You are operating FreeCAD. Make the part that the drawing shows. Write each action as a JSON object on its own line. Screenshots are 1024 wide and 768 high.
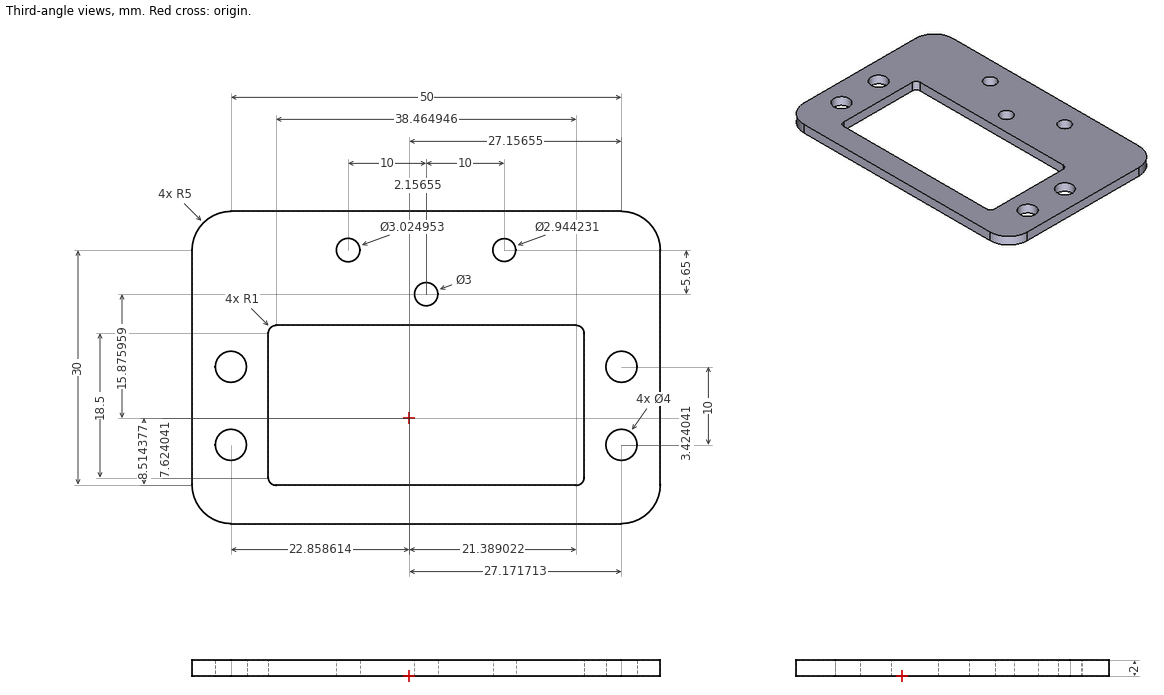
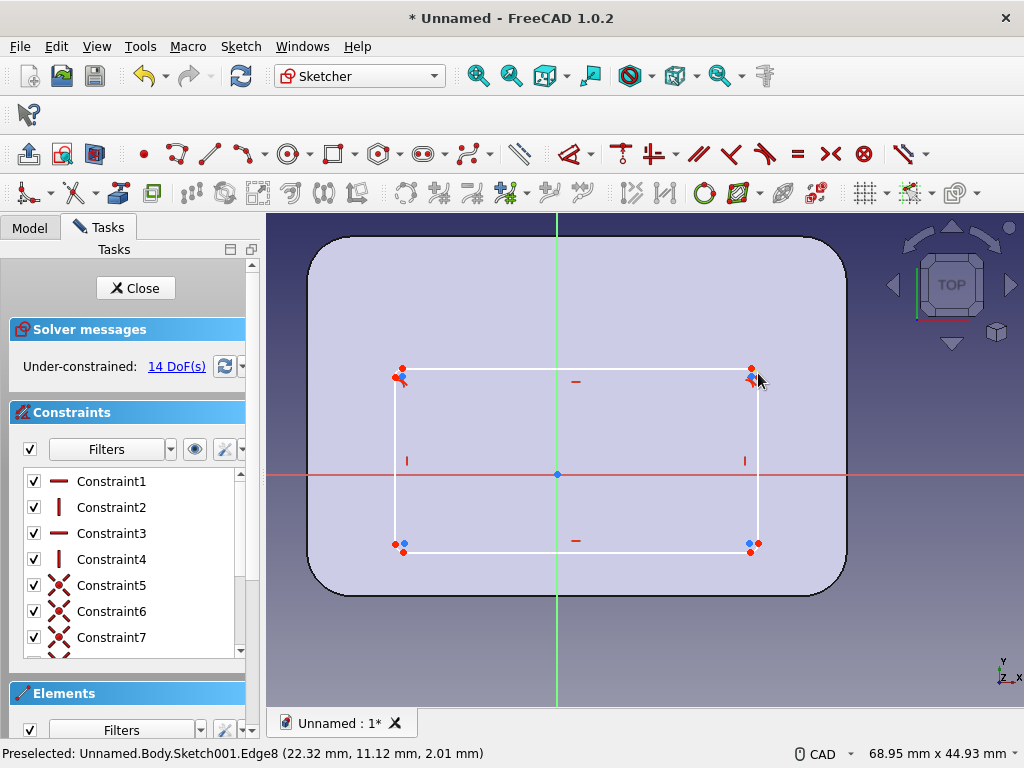
{"action": "left_click", "coordinate": [395, 428]}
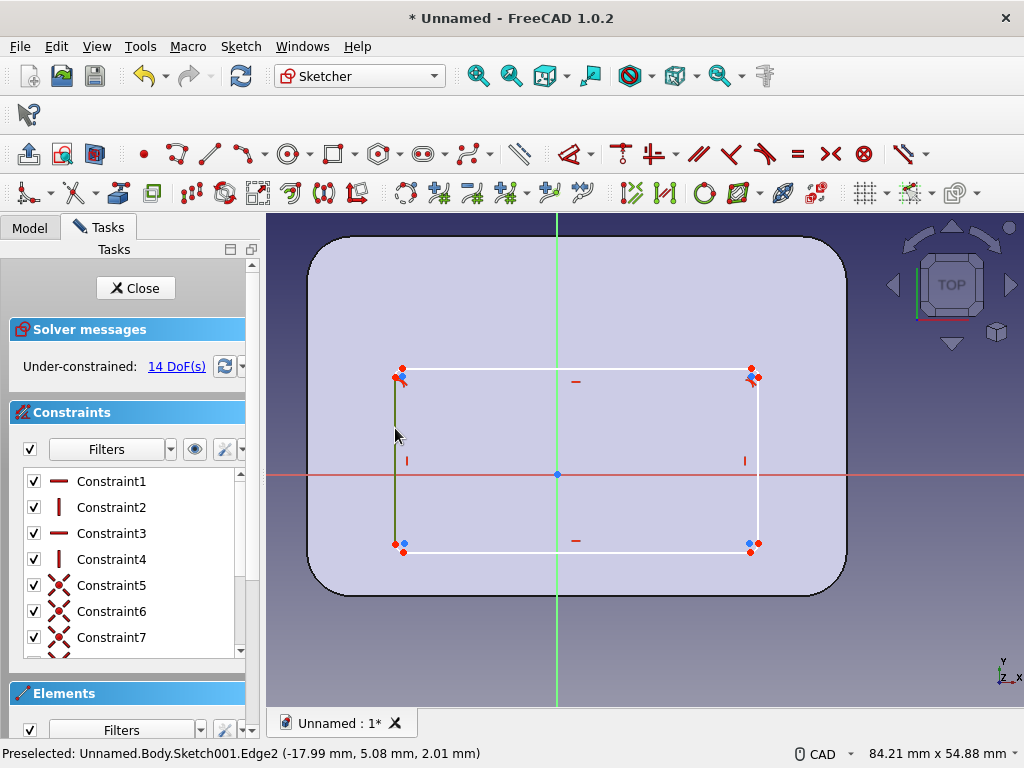
{"action": "scroll", "coordinate": [397, 372], "scroll_direction": "up", "scroll_amount": 4}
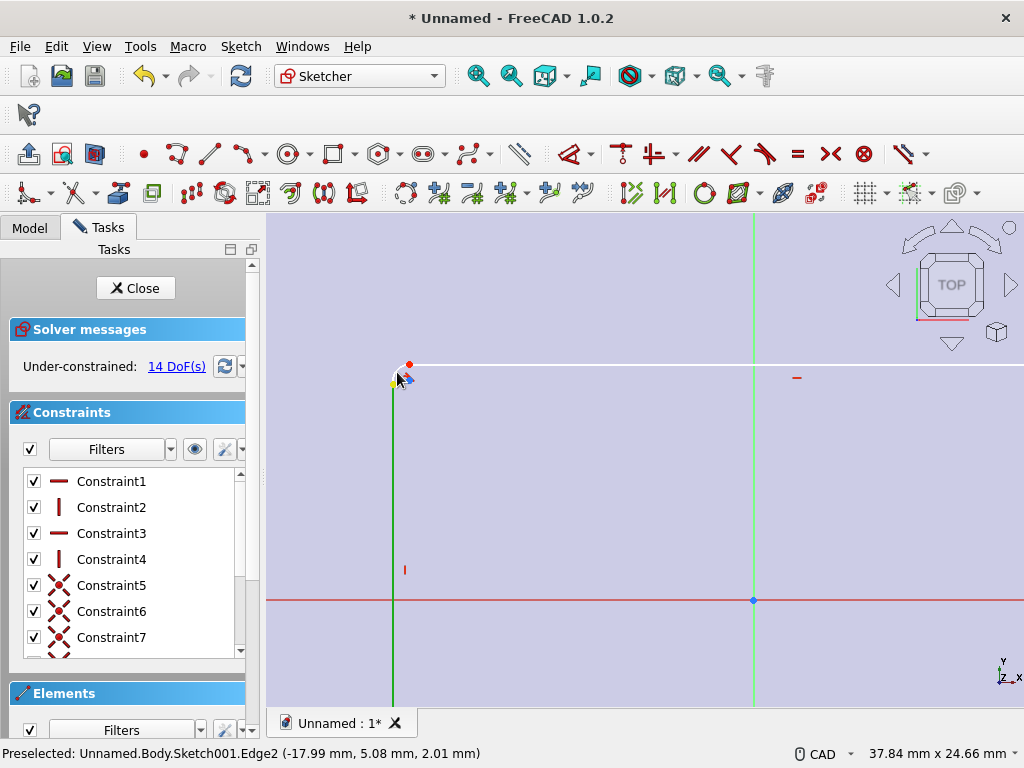
{"action": "left_click", "coordinate": [397, 371]}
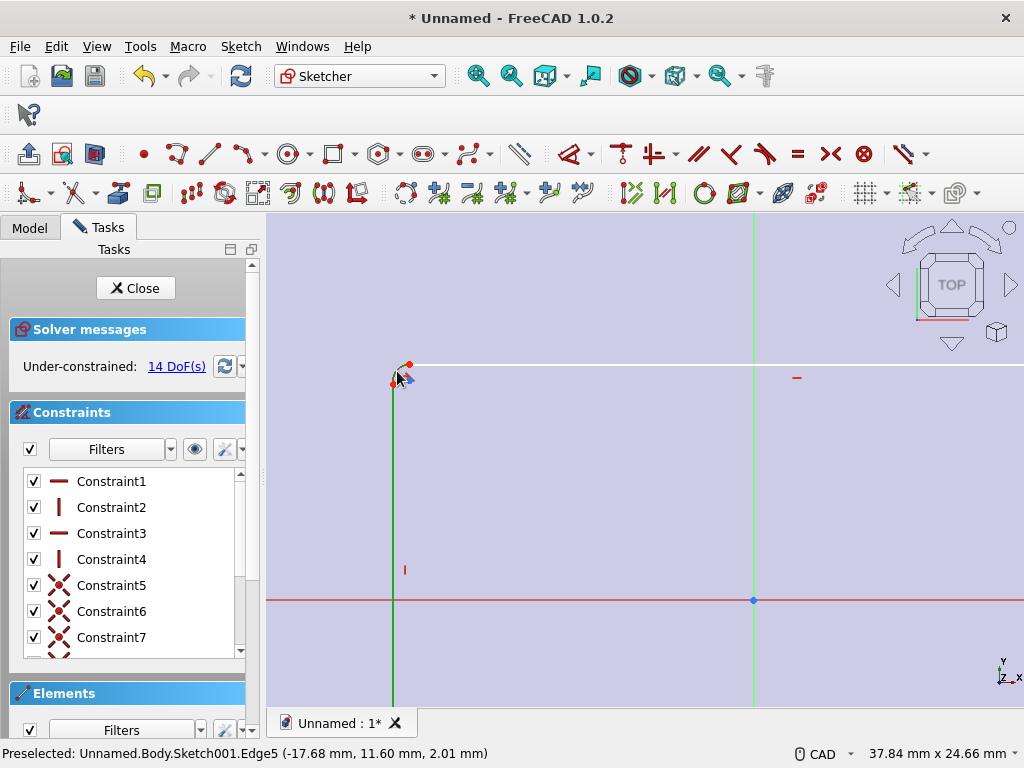
{"action": "left_click", "coordinate": [765, 154]}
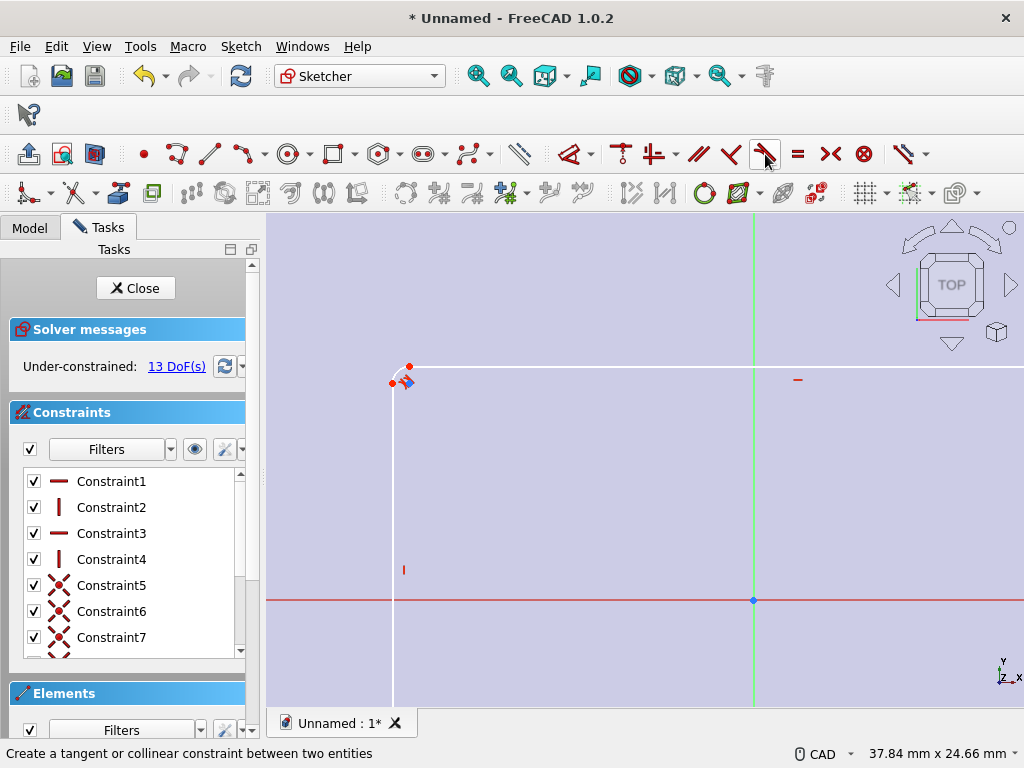
{"action": "left_click", "coordinate": [393, 495]}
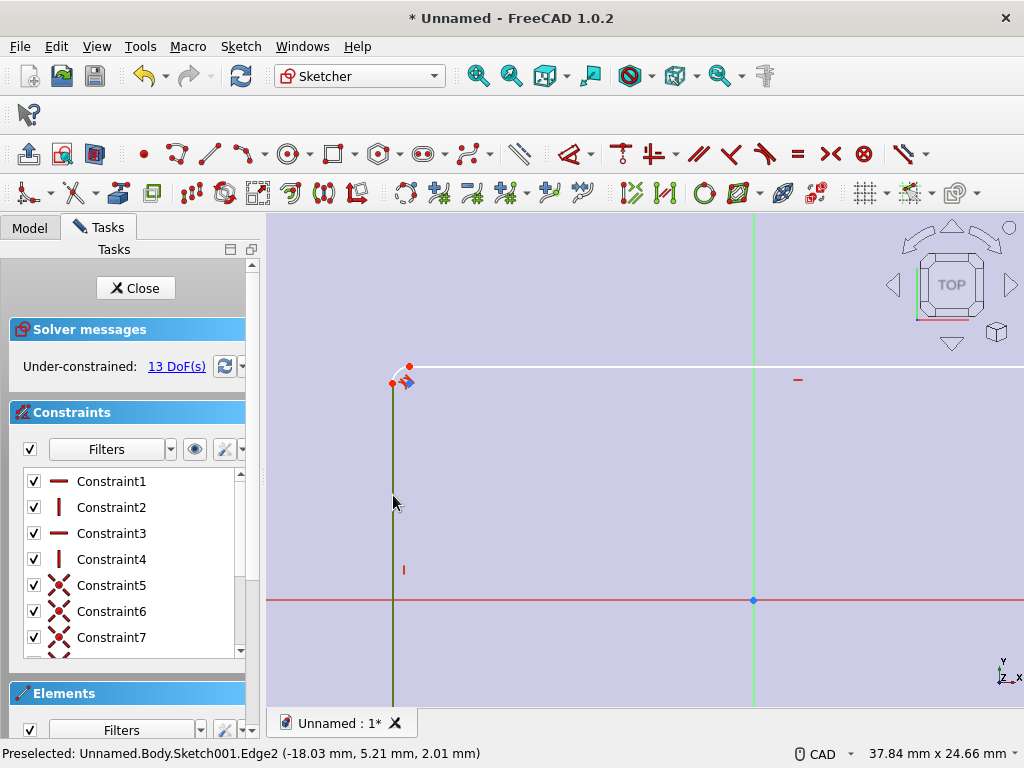
{"action": "scroll", "coordinate": [397, 372], "scroll_direction": "down", "scroll_amount": 4}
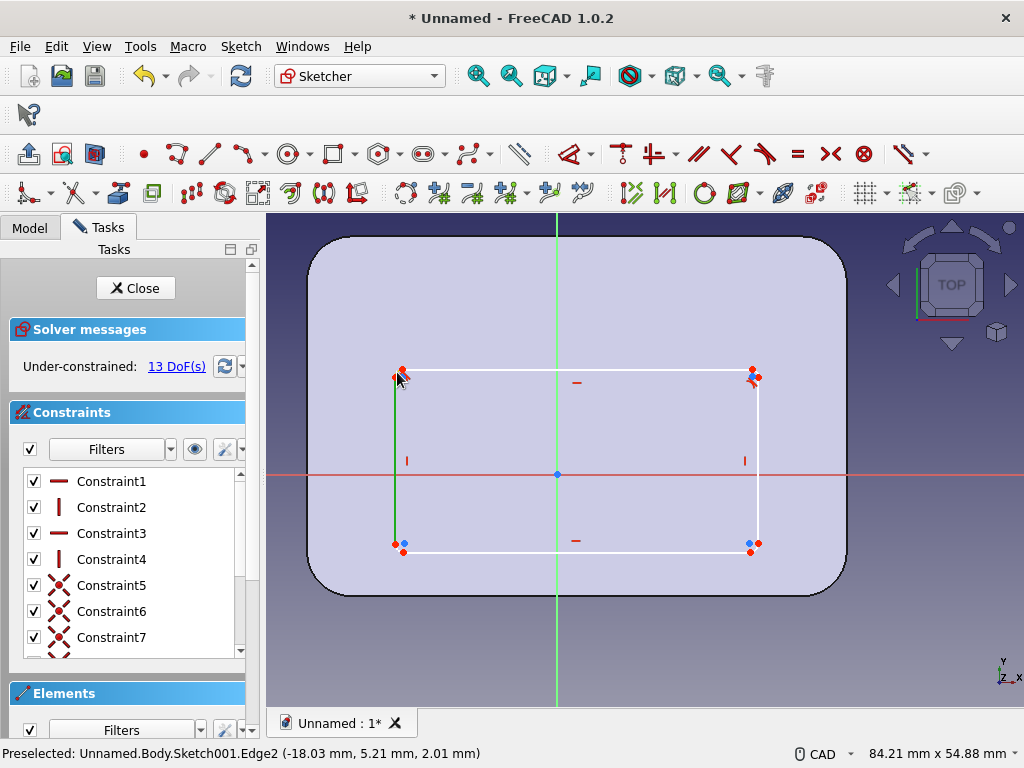
{"action": "scroll", "coordinate": [398, 550], "scroll_direction": "up", "scroll_amount": 5}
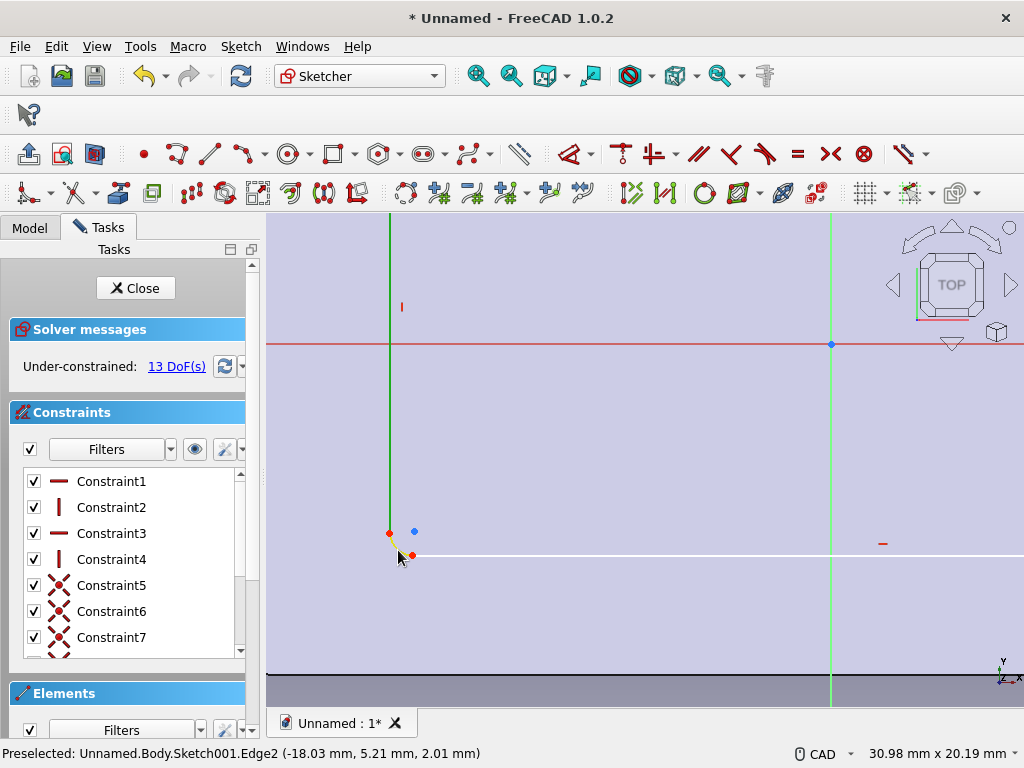
{"action": "left_click", "coordinate": [397, 549]}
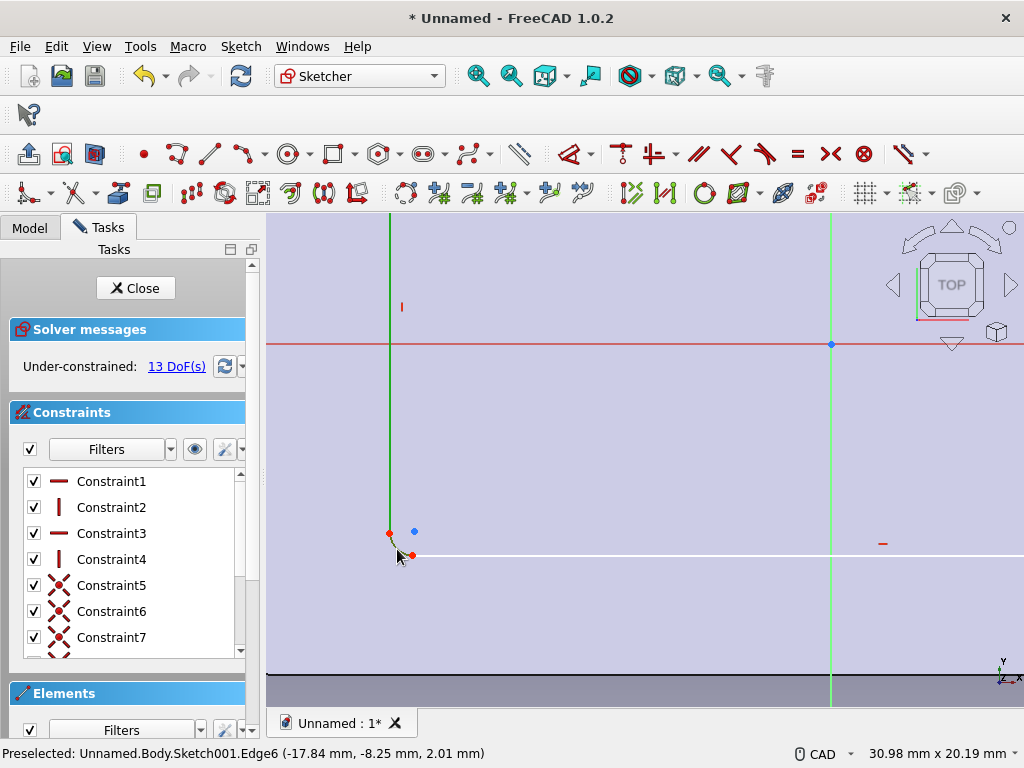
{"action": "left_click", "coordinate": [765, 154]}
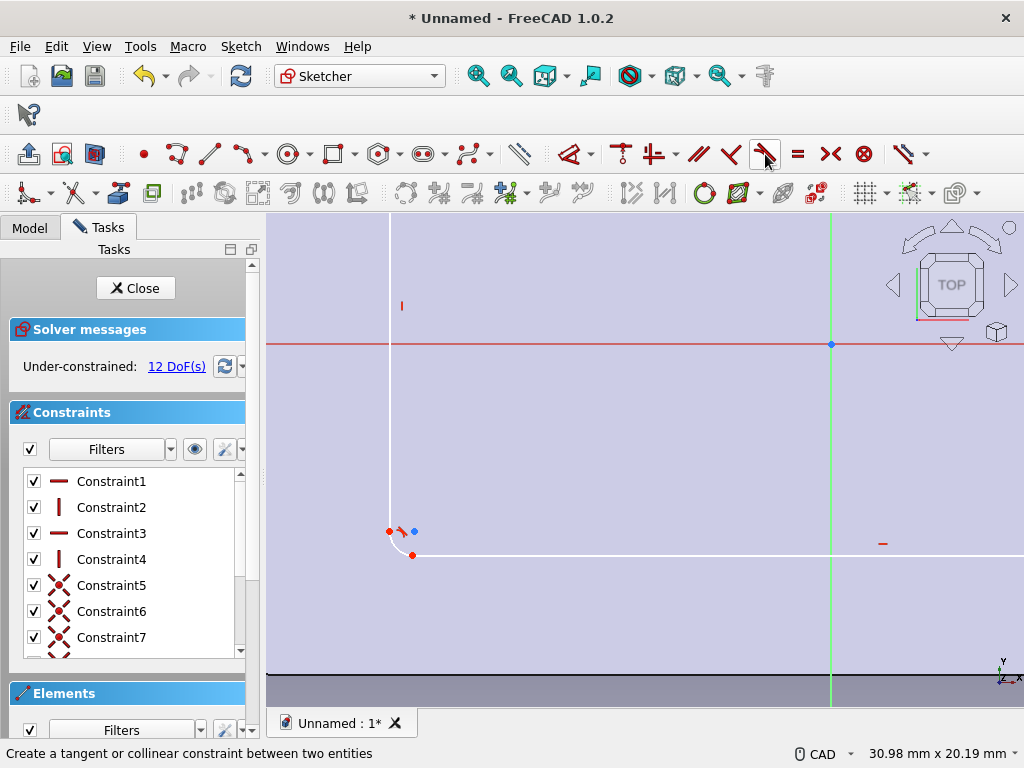
{"action": "left_click", "coordinate": [695, 556]}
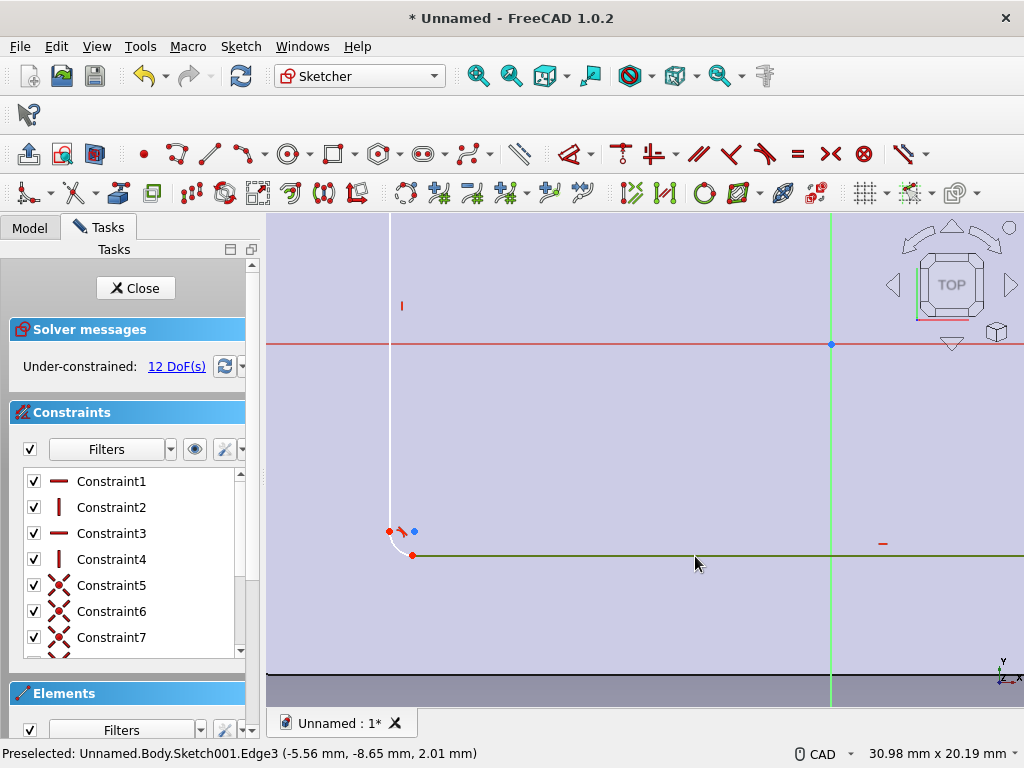
{"action": "scroll", "coordinate": [392, 542], "scroll_direction": "up", "scroll_amount": 2}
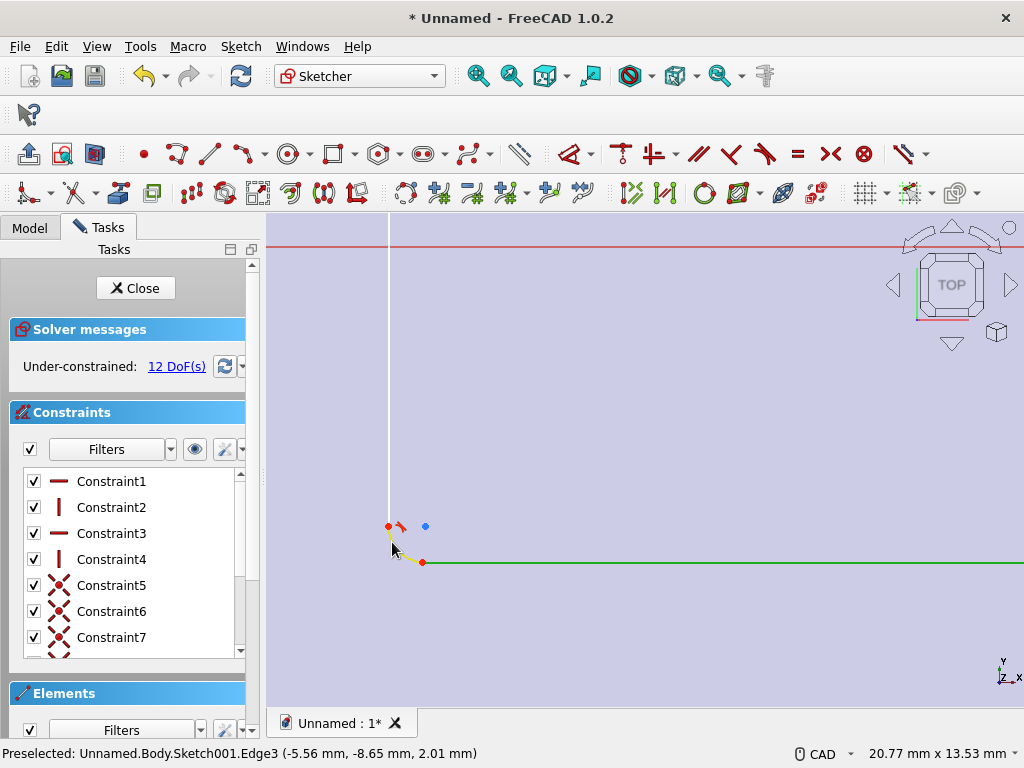
{"action": "left_click", "coordinate": [392, 542]}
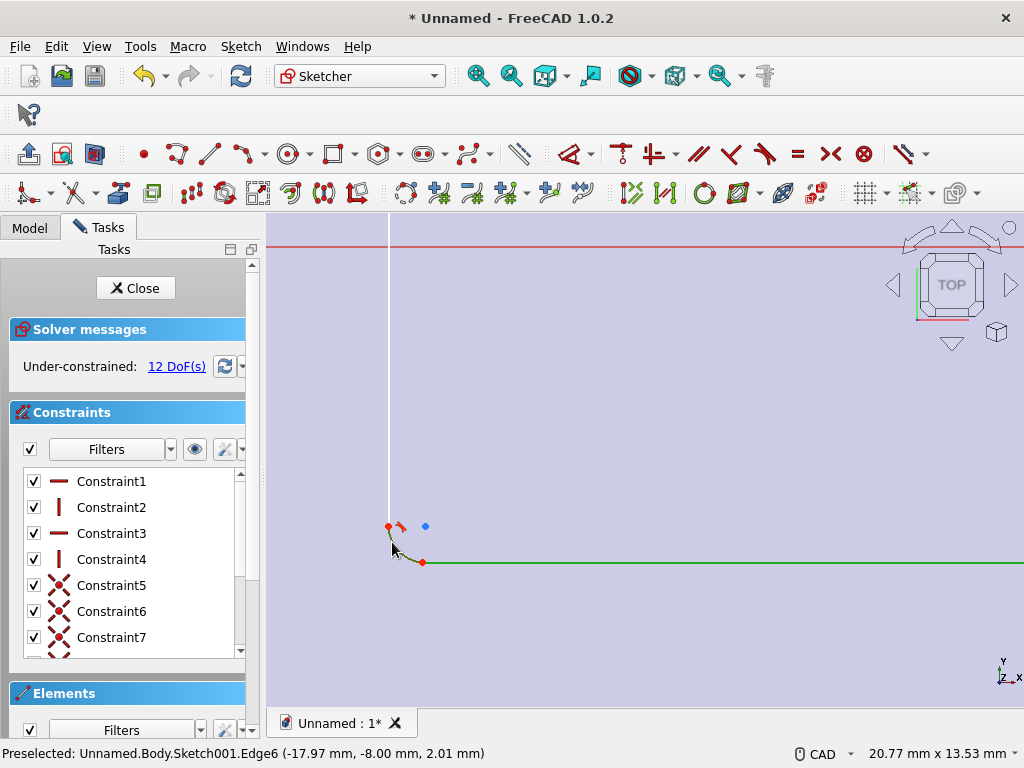
{"action": "left_click", "coordinate": [765, 154]}